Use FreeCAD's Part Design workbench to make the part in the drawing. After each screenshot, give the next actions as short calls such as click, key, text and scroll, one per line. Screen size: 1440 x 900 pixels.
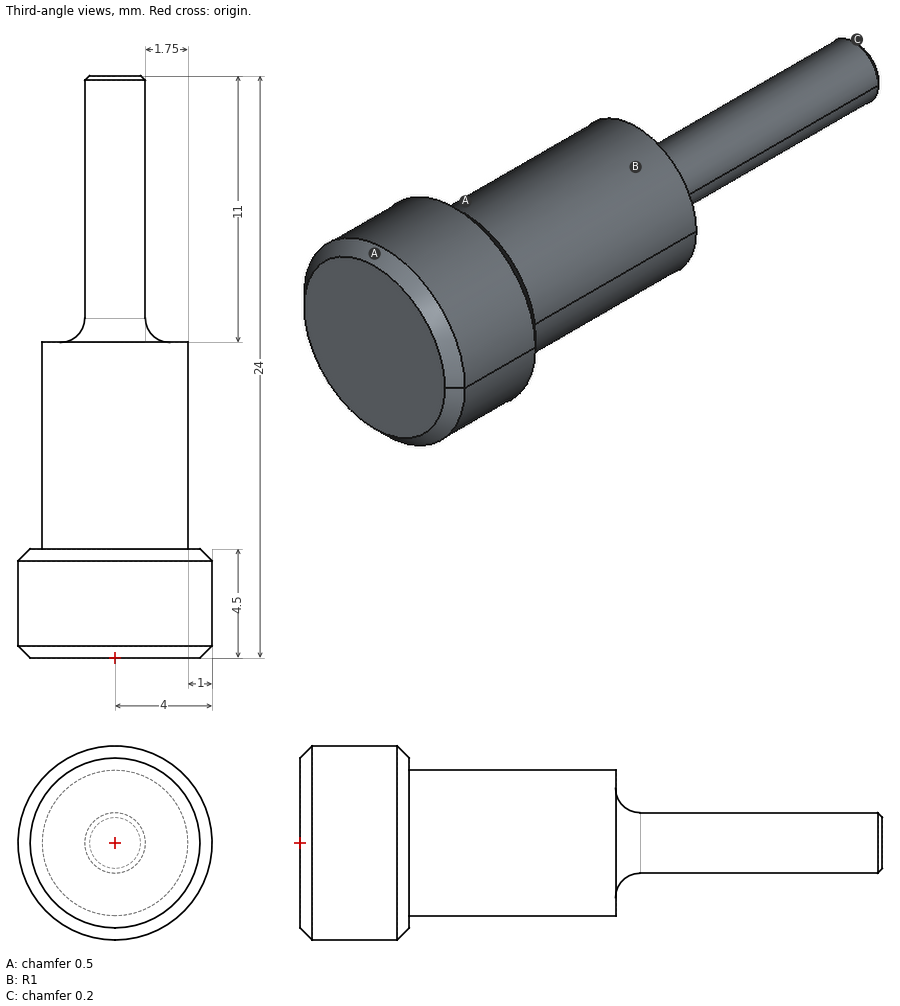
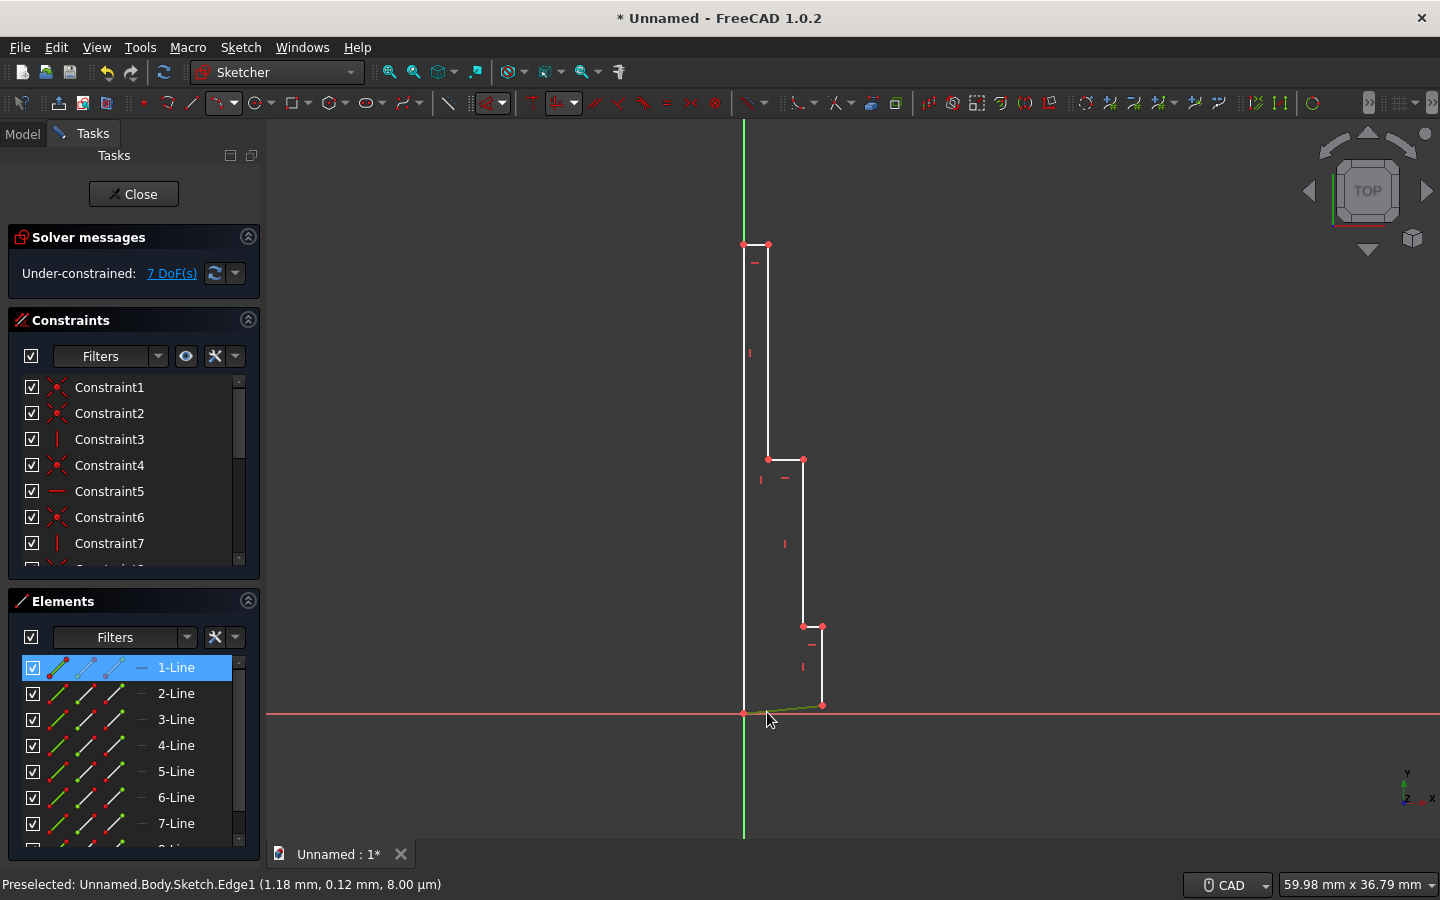
key(h)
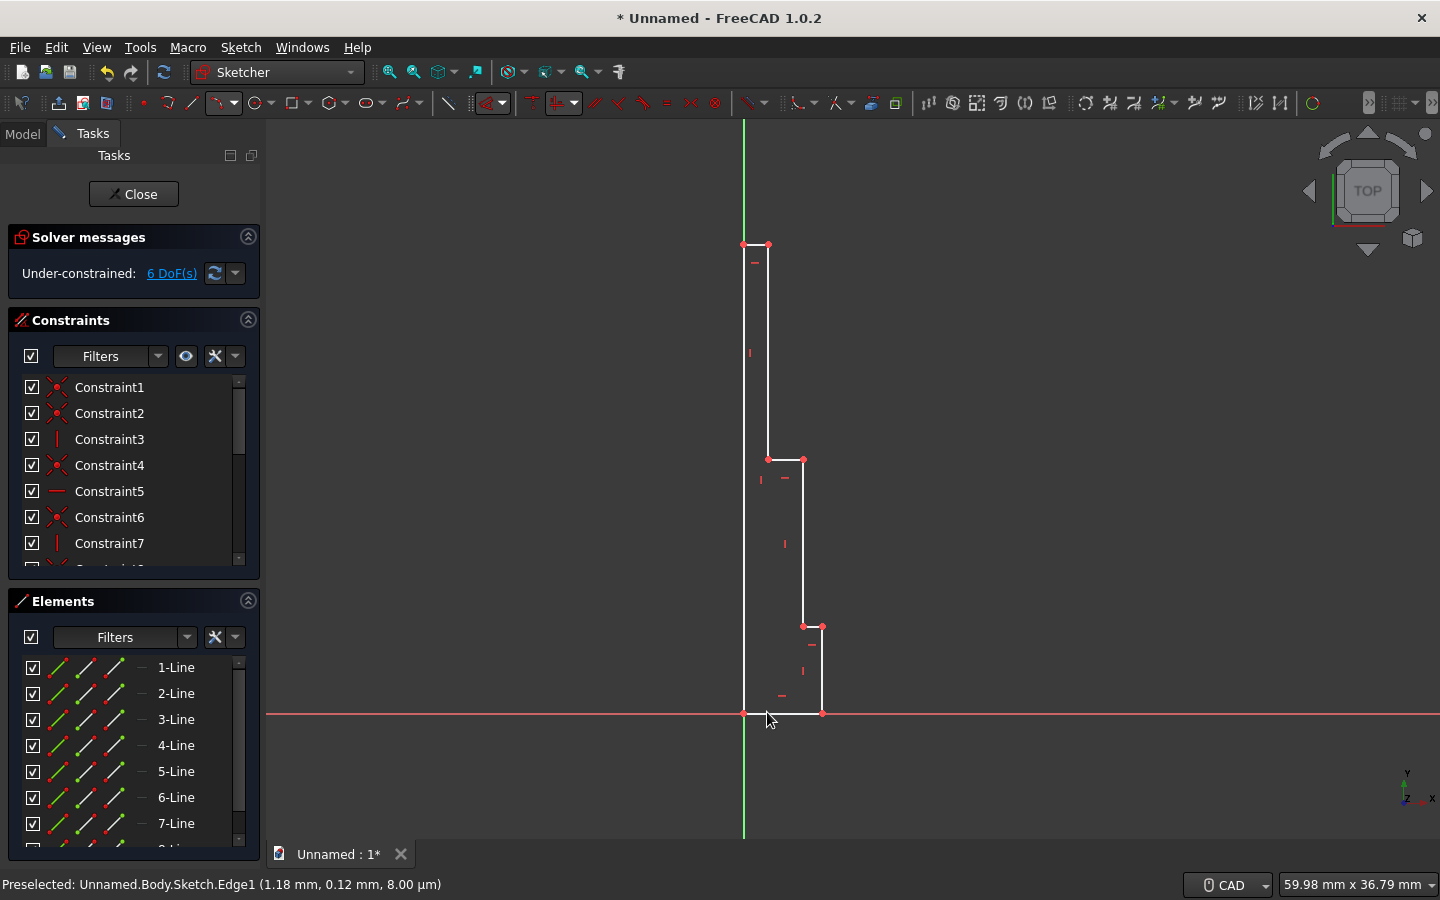
click(486, 104)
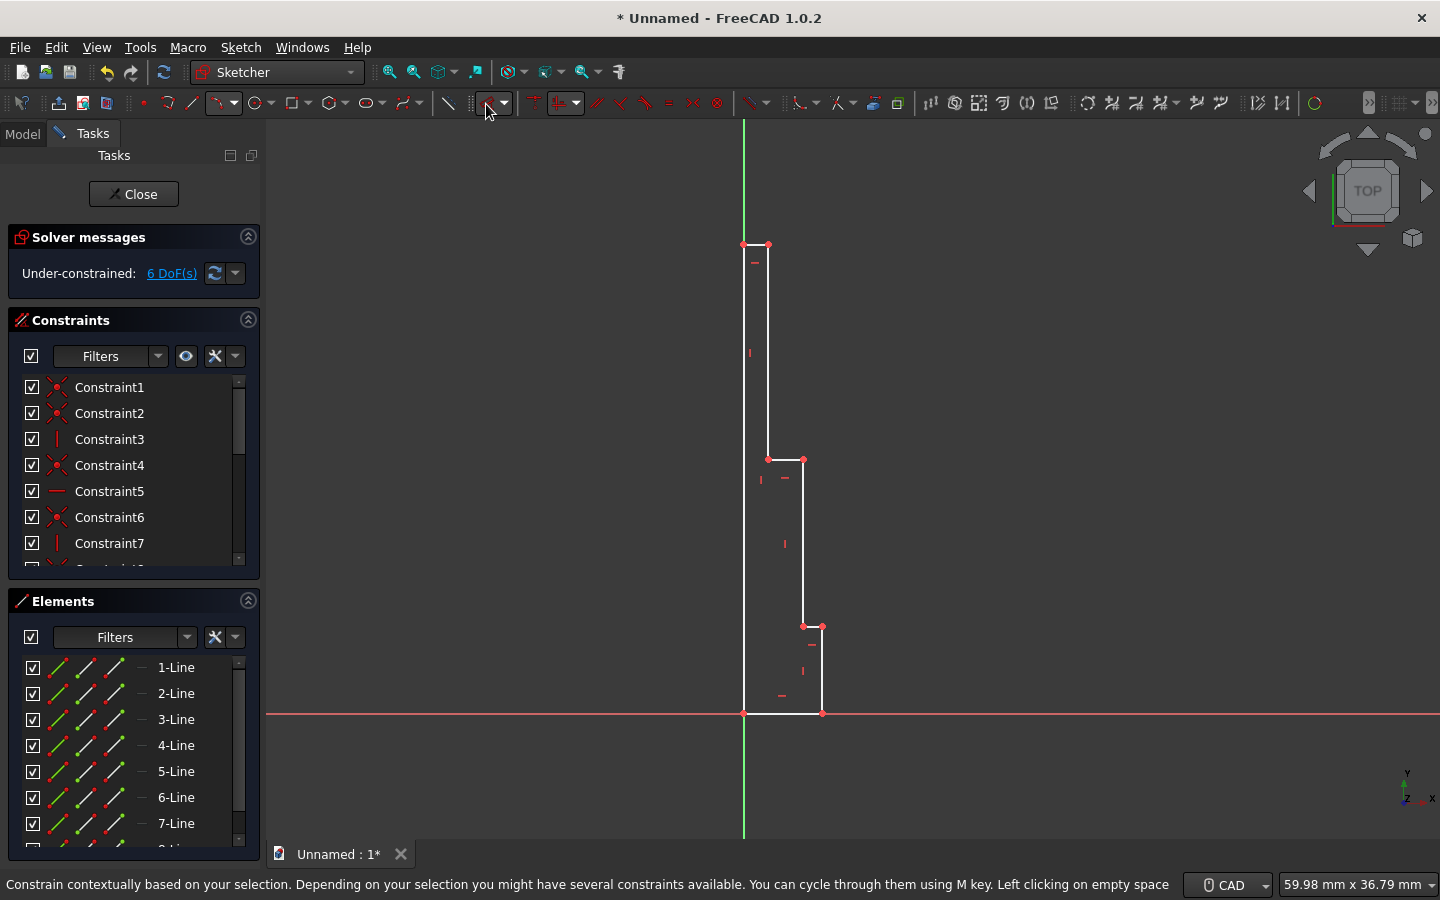
click(767, 714)
click(783, 748)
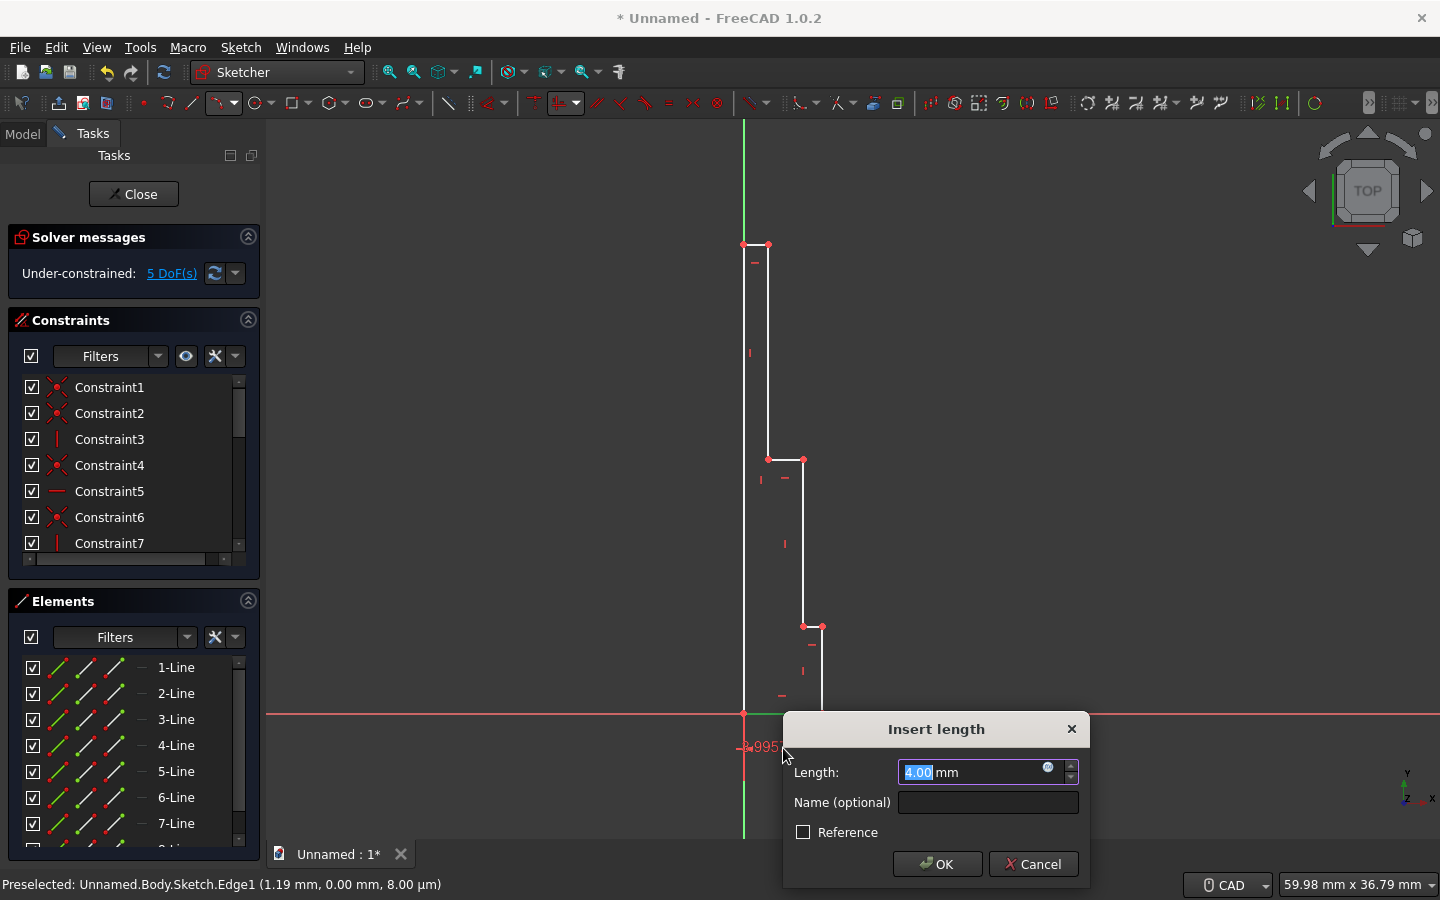
text(4)
key(Return)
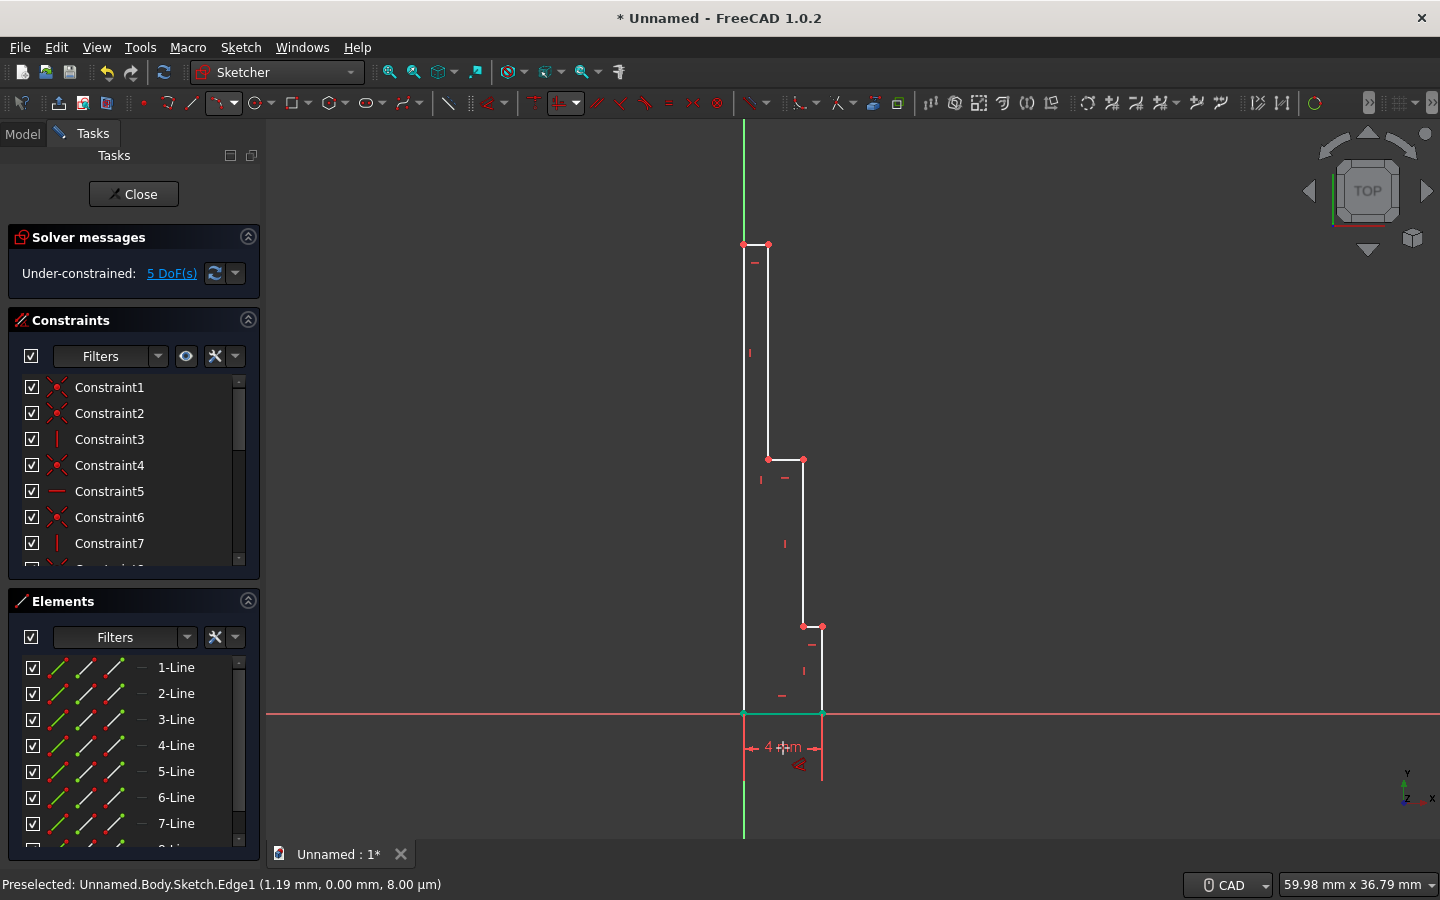
scroll(813, 627, up, 4)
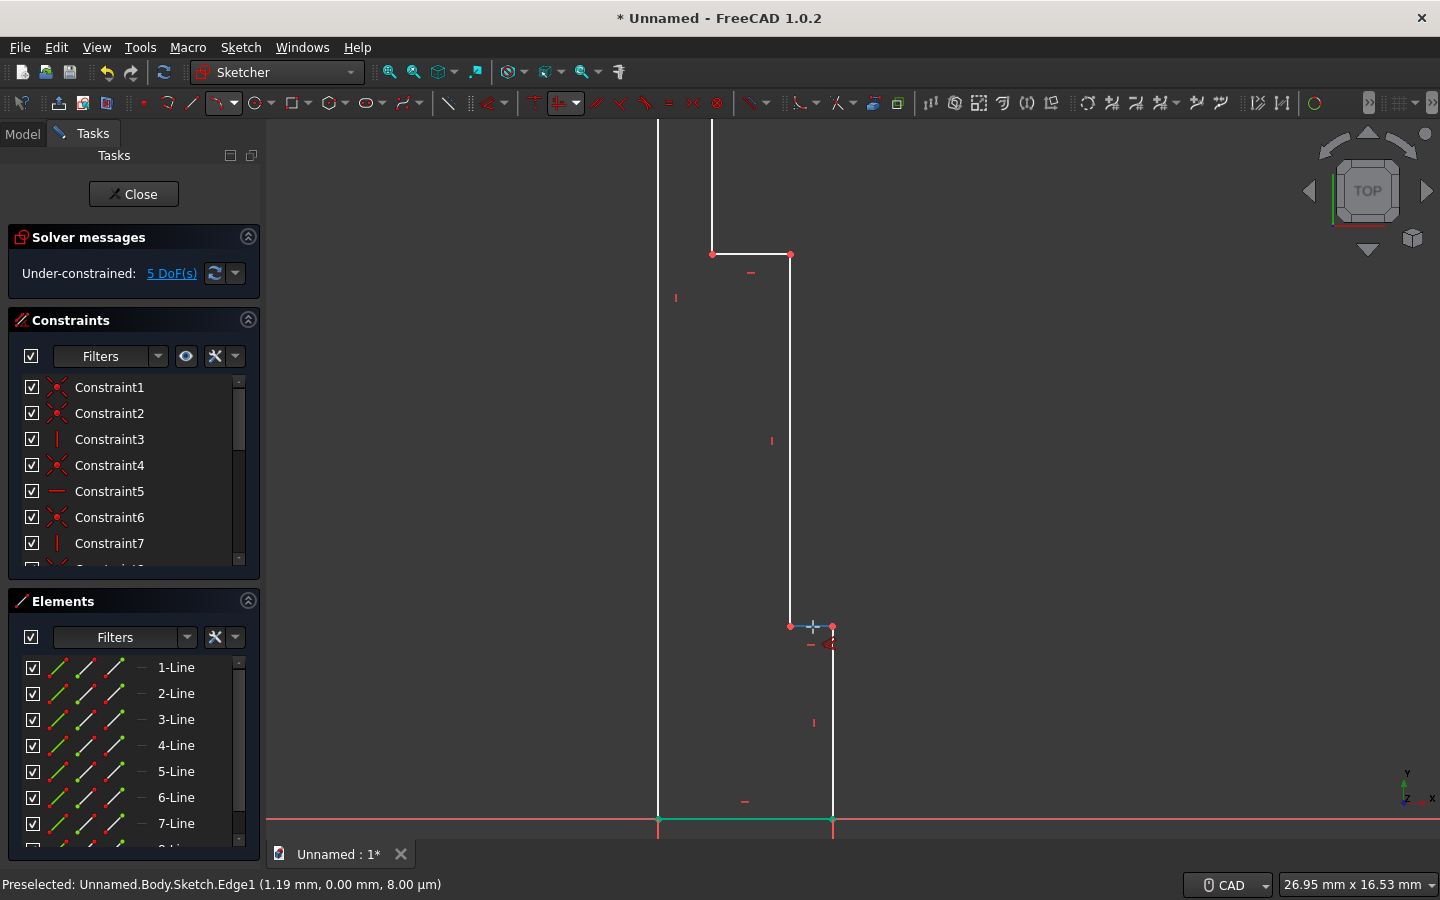
click(811, 626)
click(811, 660)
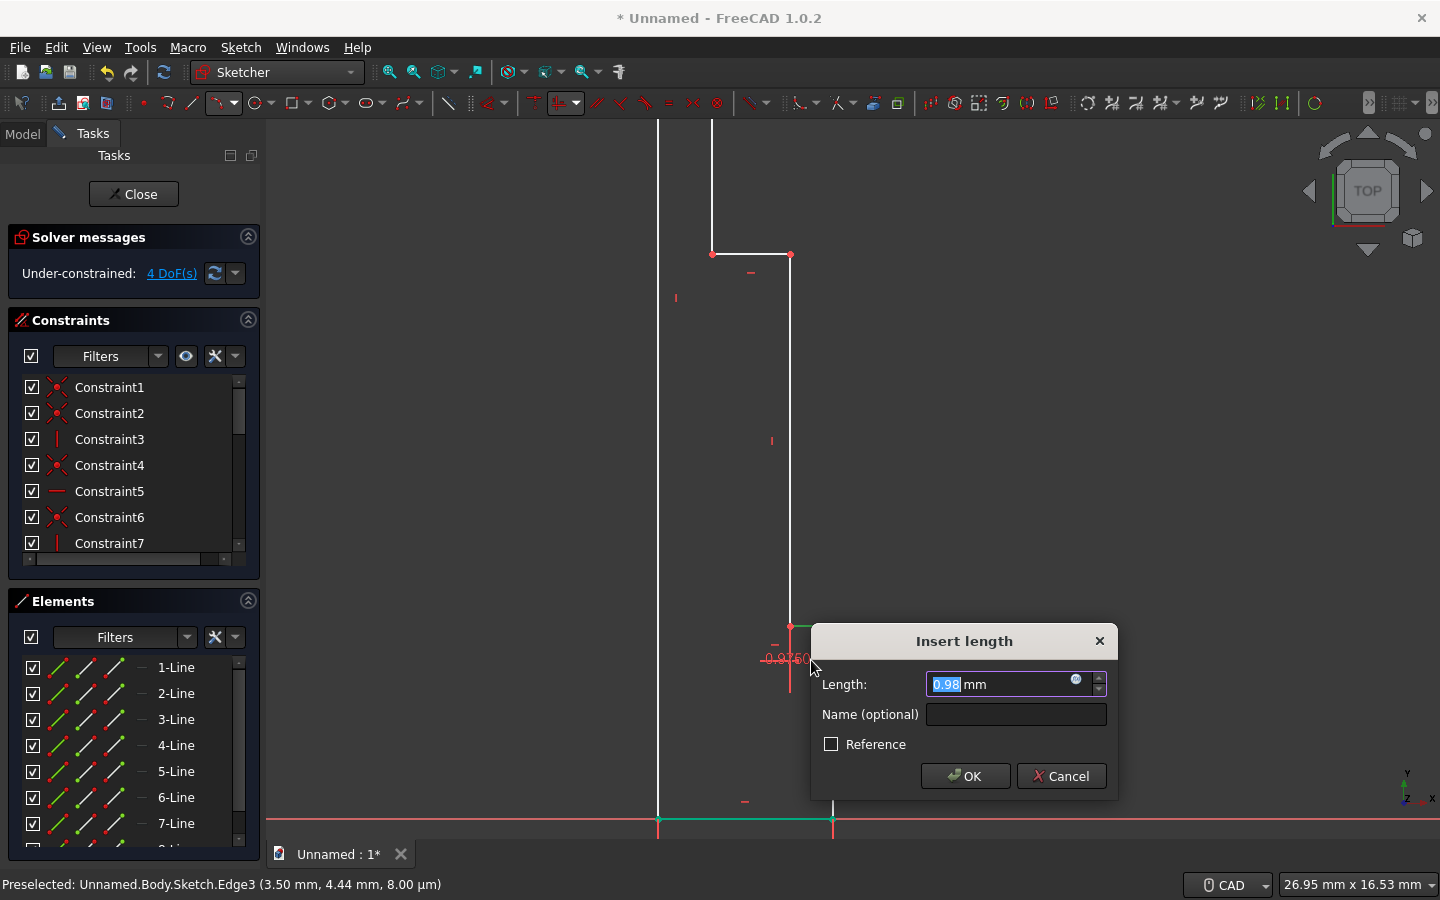
text(1)
key(Return)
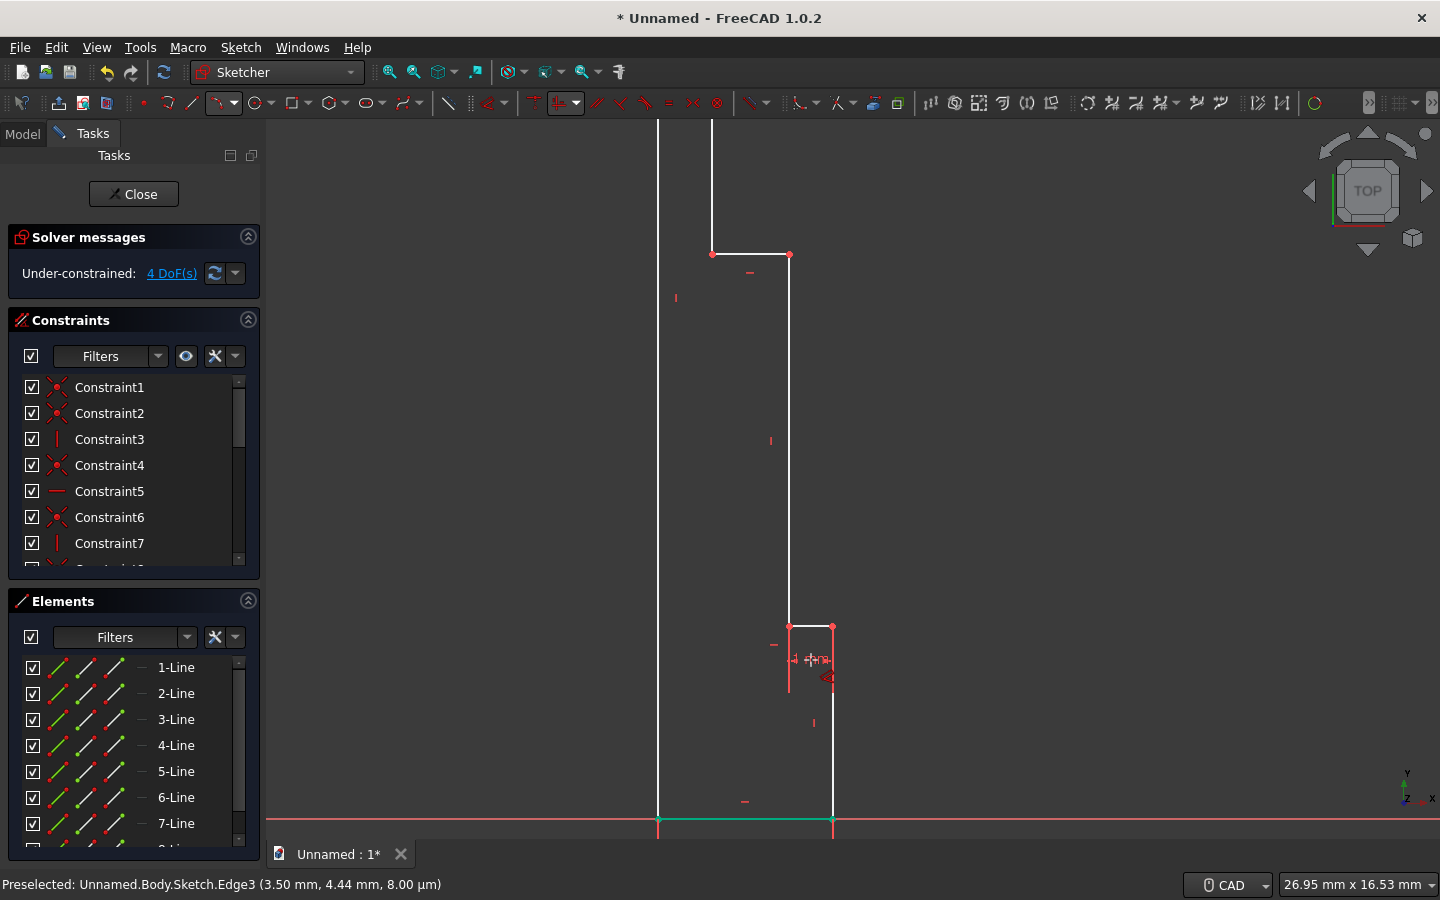
click(712, 159)
click(678, 201)